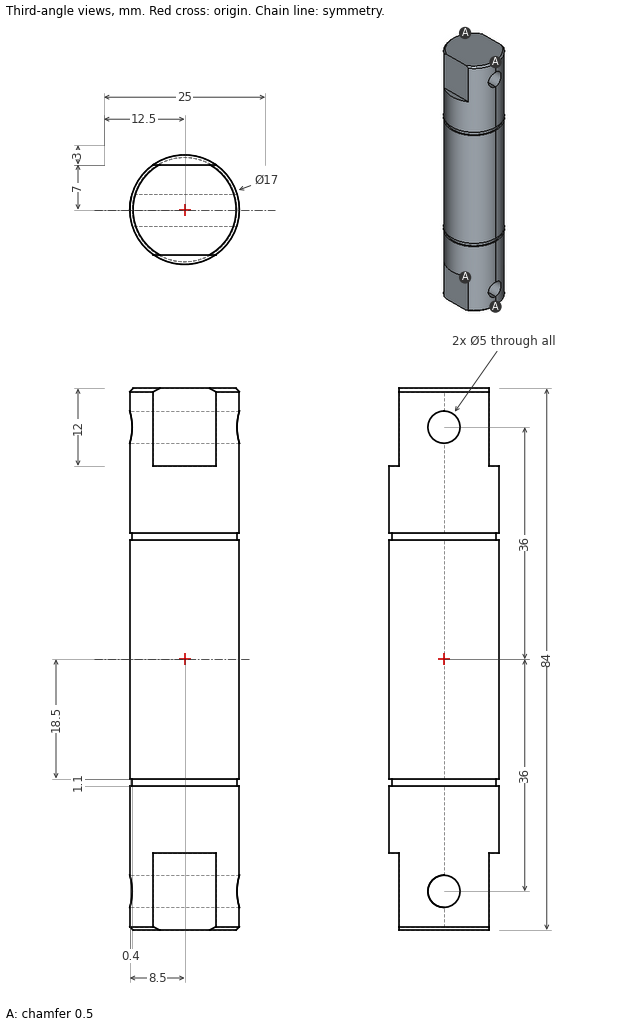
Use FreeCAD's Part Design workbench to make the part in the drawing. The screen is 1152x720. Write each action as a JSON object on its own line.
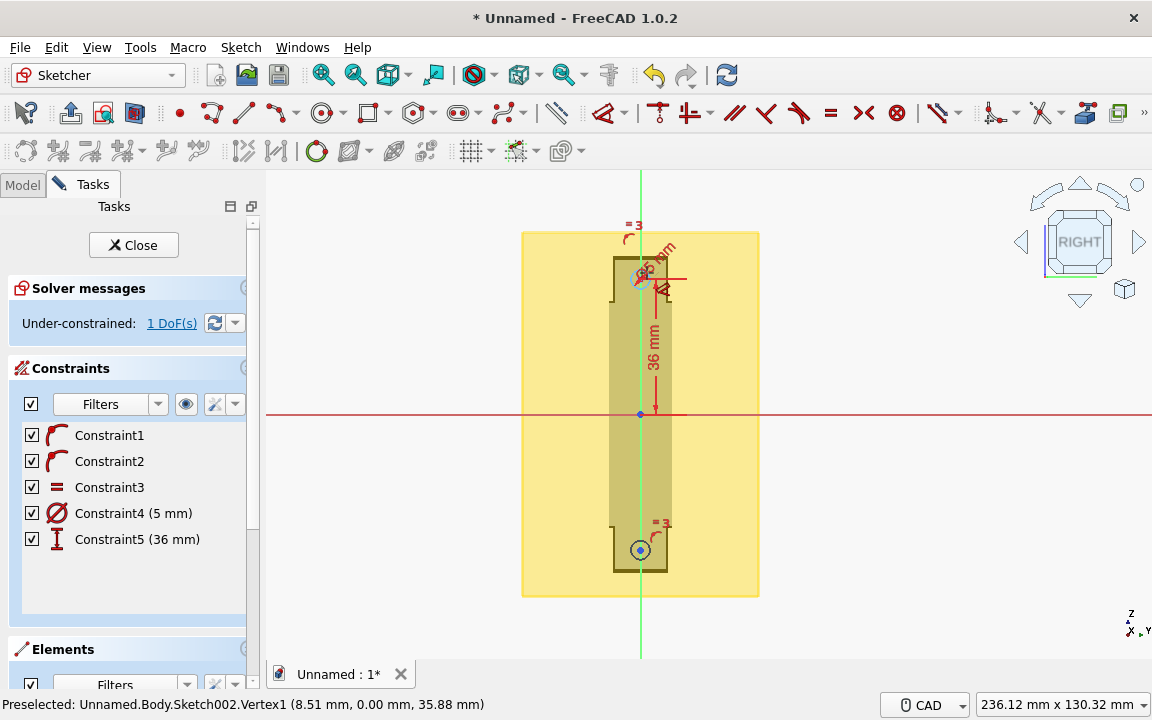
{"action": "left_click", "coordinate": [641, 550]}
{"action": "left_click", "coordinate": [675, 482]}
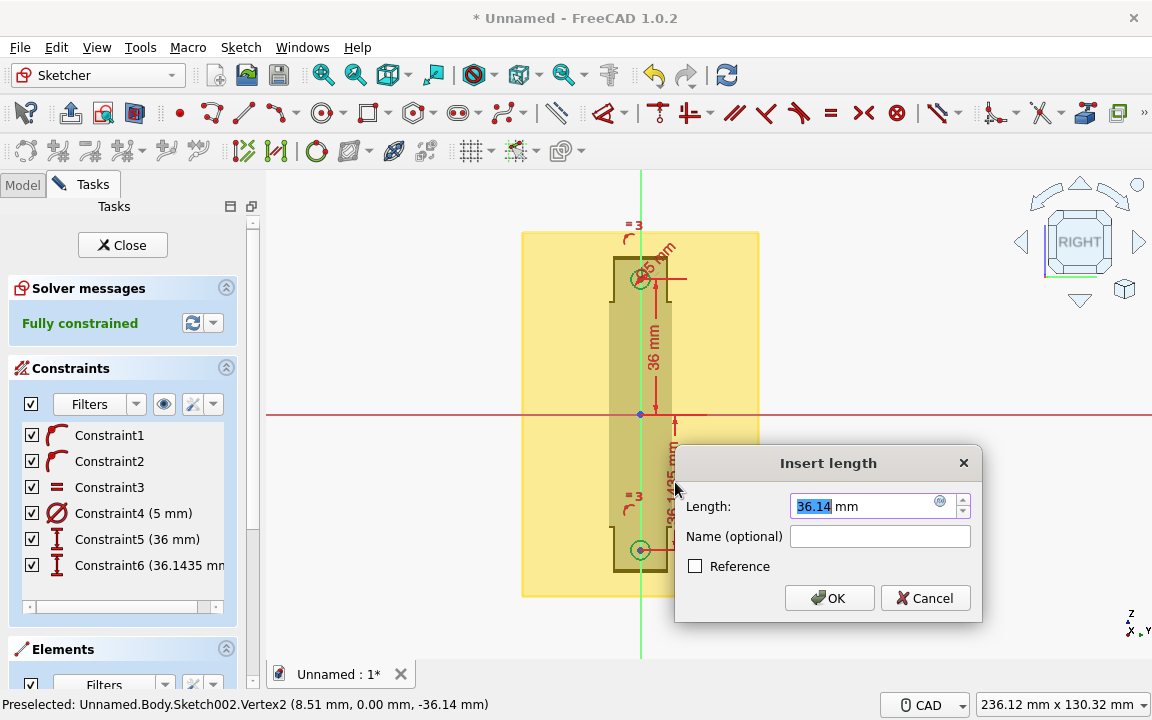
{"action": "type", "text": "36"}
{"action": "key", "text": "Return"}
{"action": "key", "text": "Escape"}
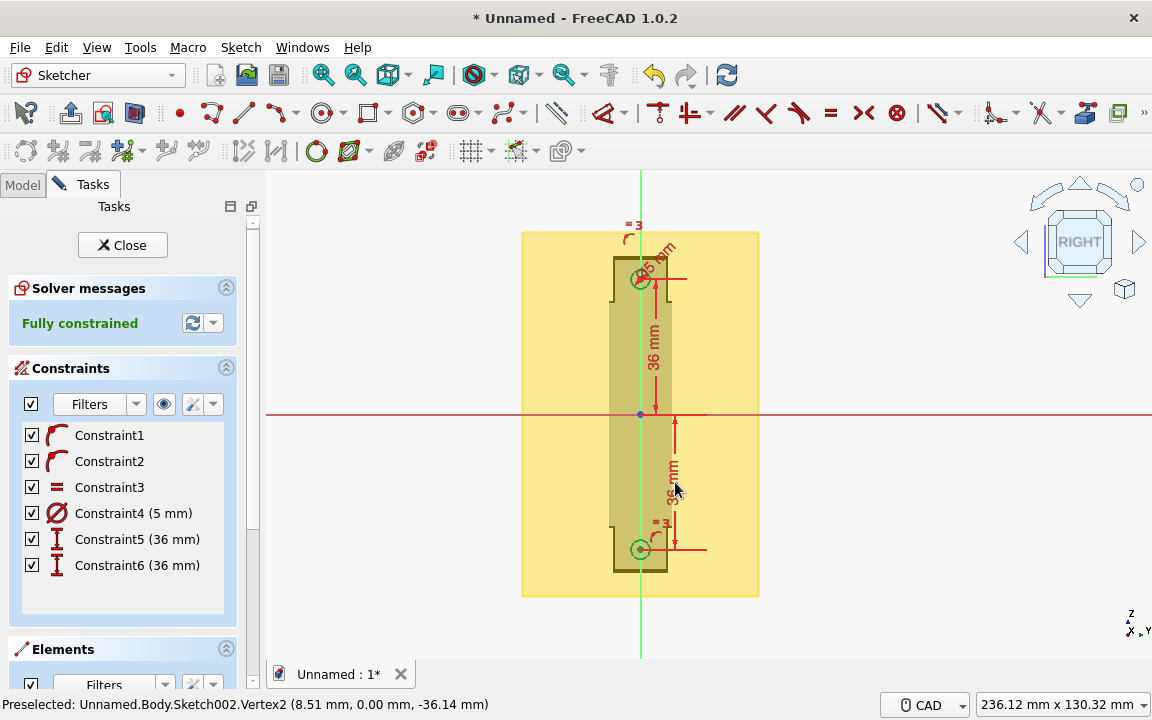
{"action": "left_click", "coordinate": [123, 245]}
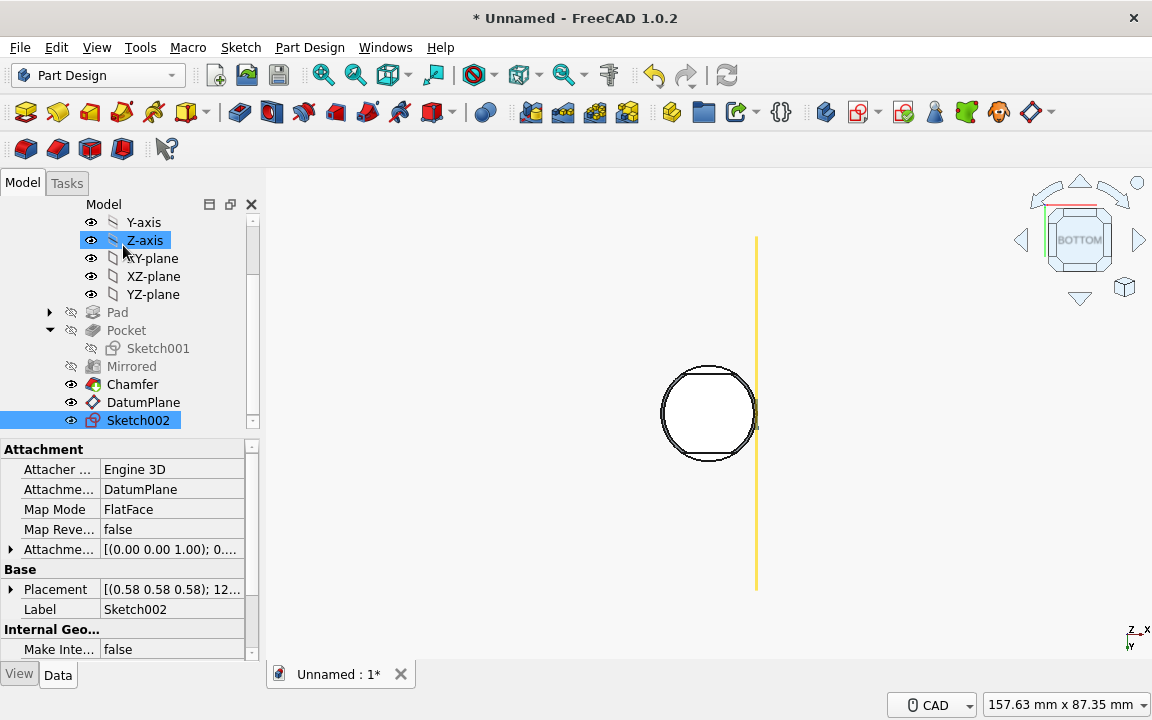
{"action": "left_click", "coordinate": [272, 112]}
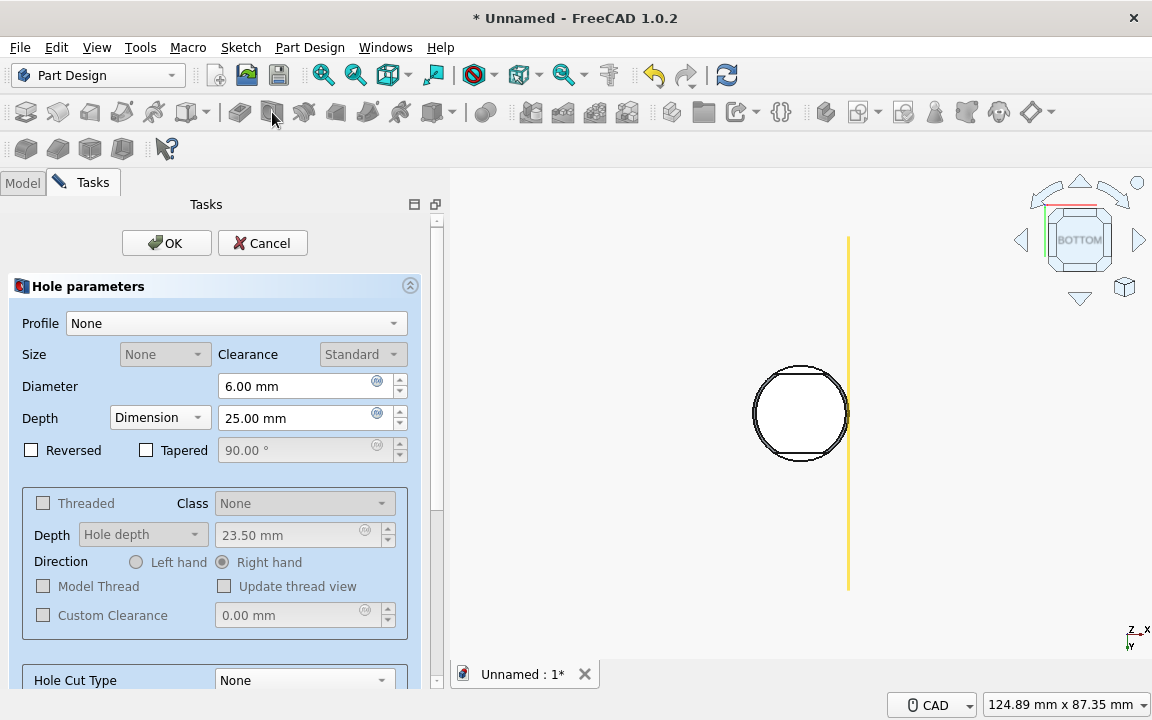
{"action": "triple_click", "coordinate": [305, 386]}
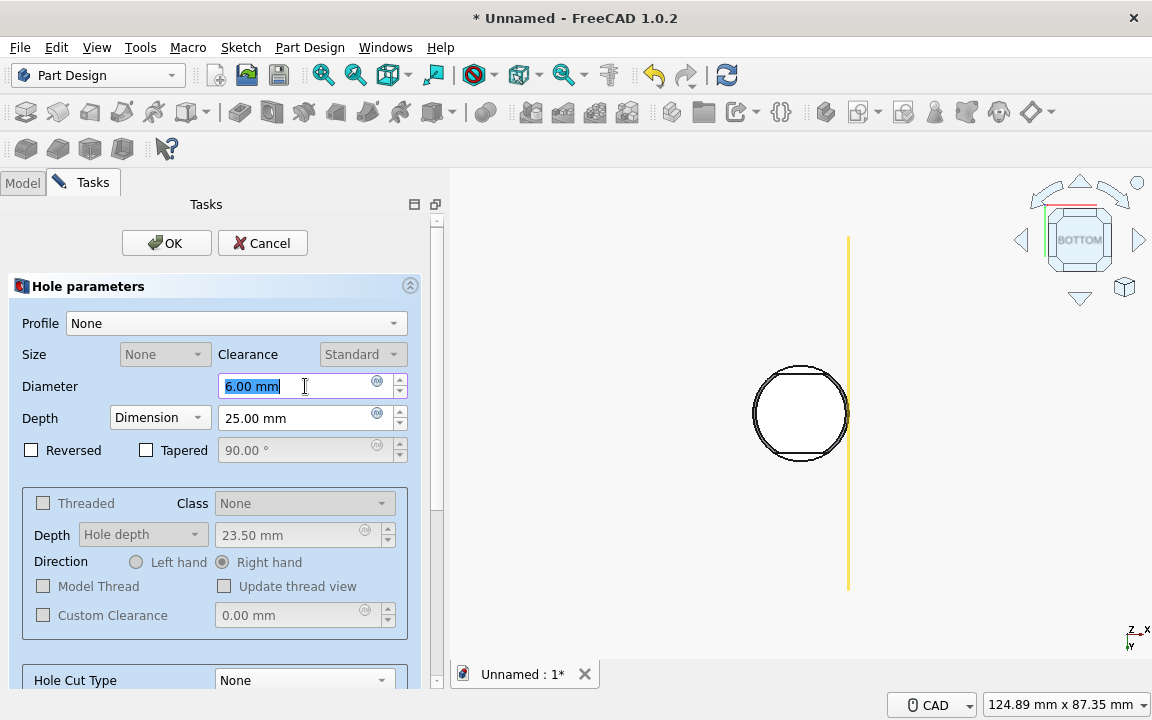
{"action": "type", "text": "5"}
{"action": "key", "text": "Tab"}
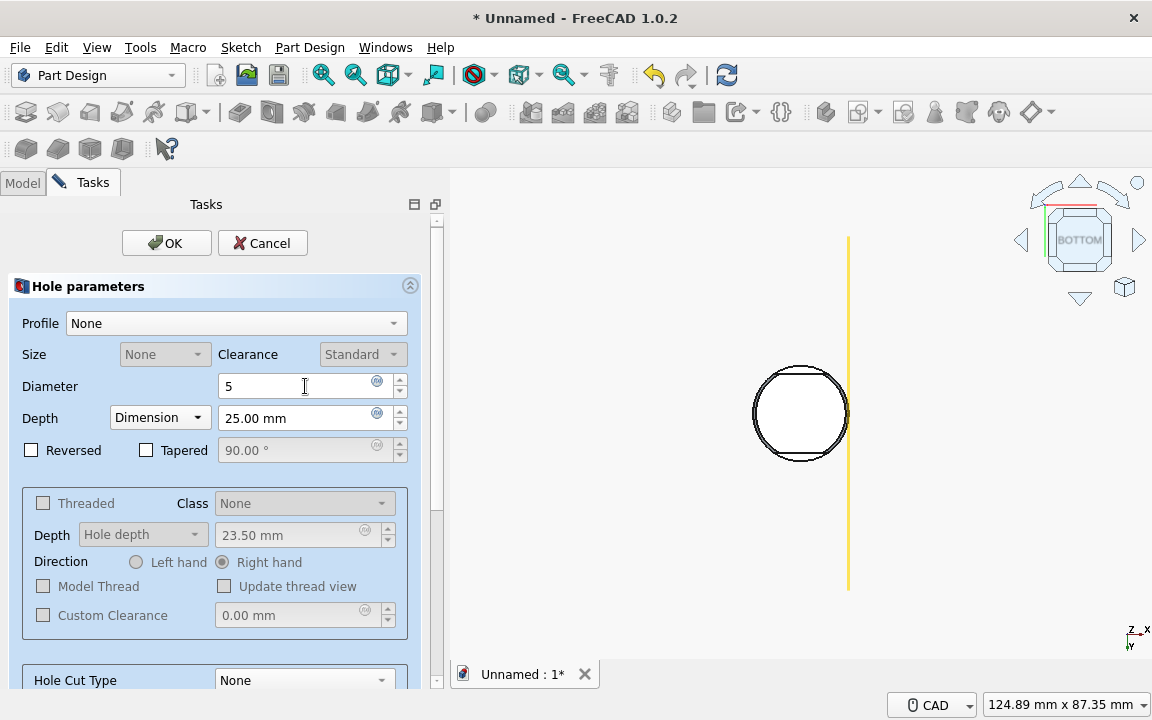
{"action": "left_click", "coordinate": [161, 418]}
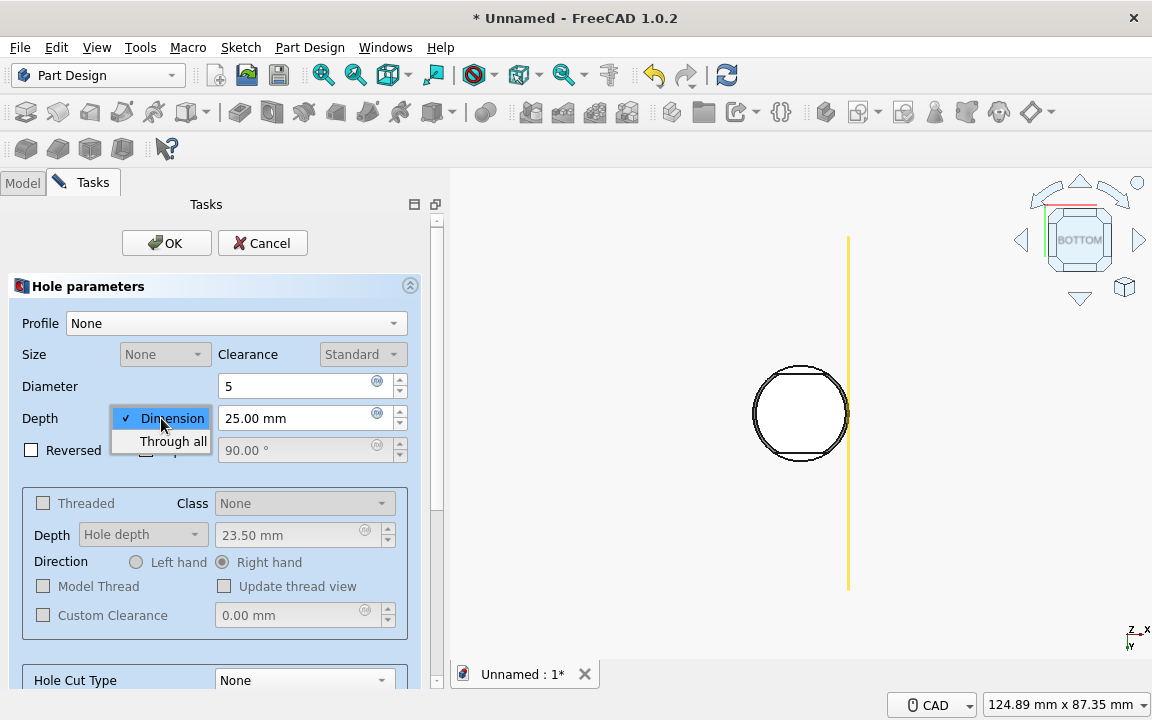
{"action": "left_click", "coordinate": [160, 442]}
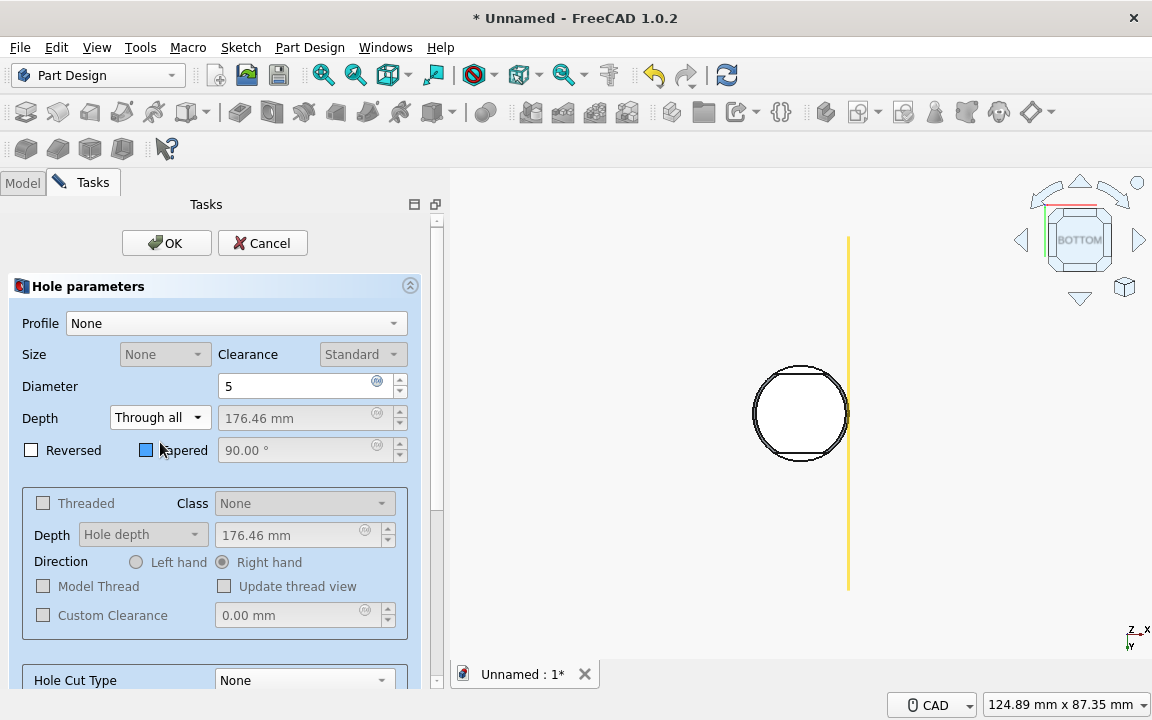
{"action": "left_click", "coordinate": [167, 243]}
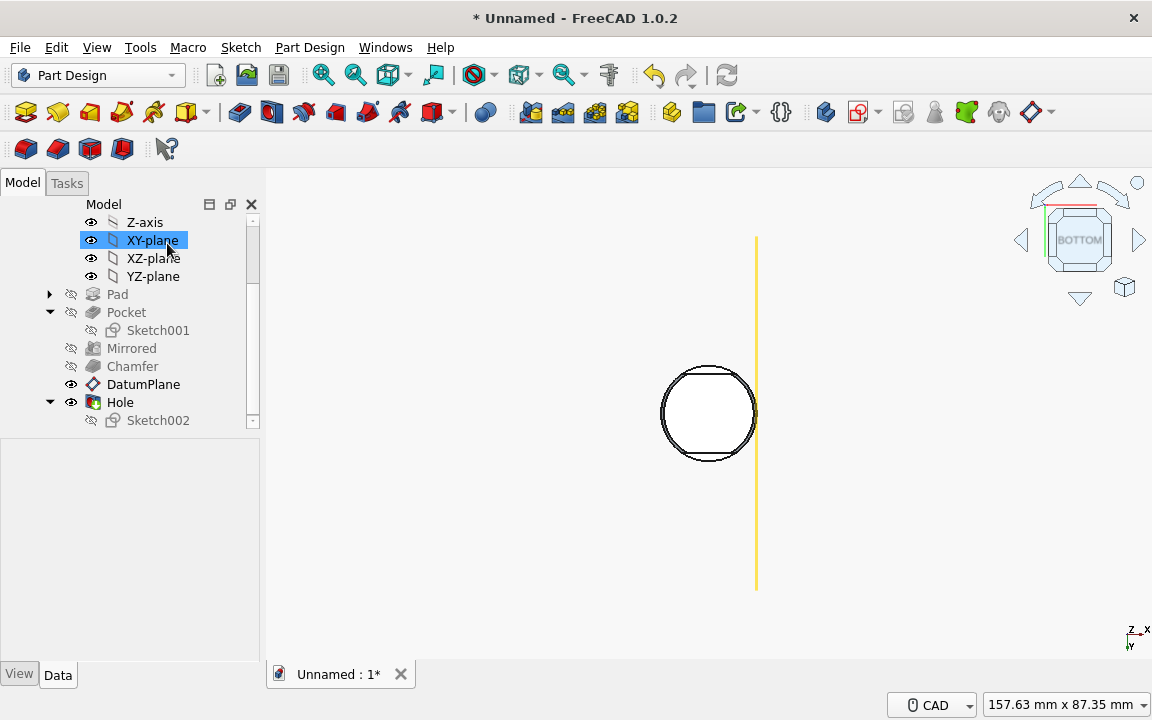
{"action": "left_click", "coordinate": [116, 384]}
{"action": "key", "text": "space"}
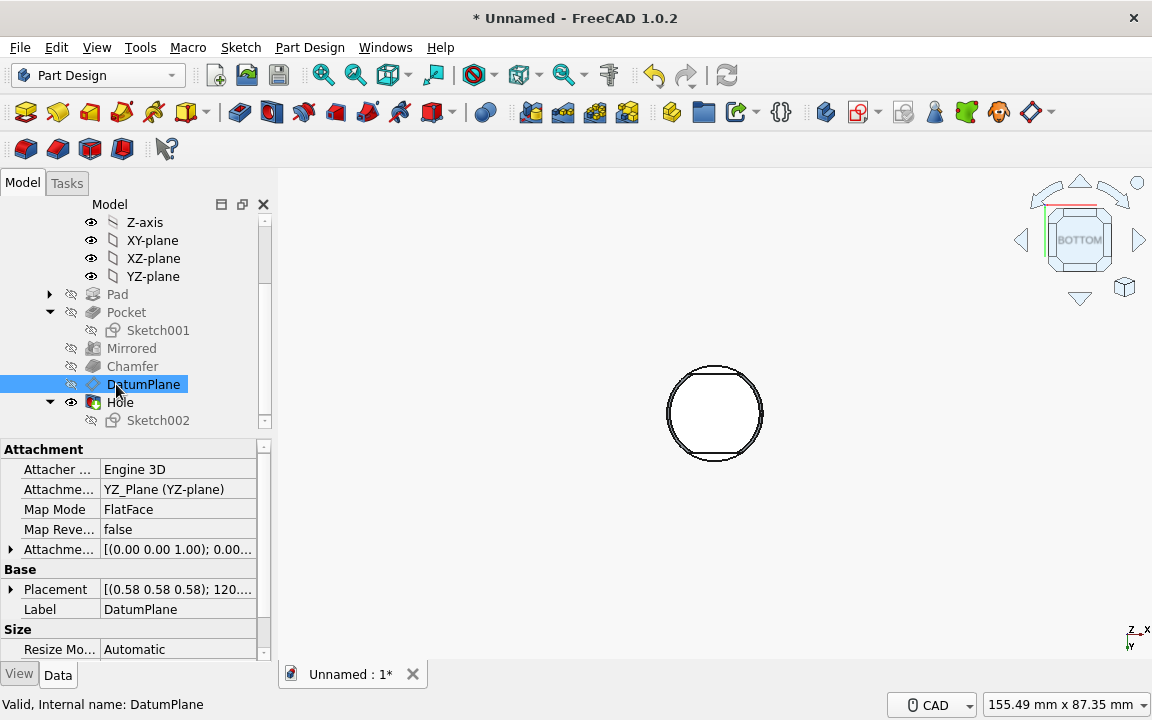
{"action": "left_click", "coordinate": [324, 76]}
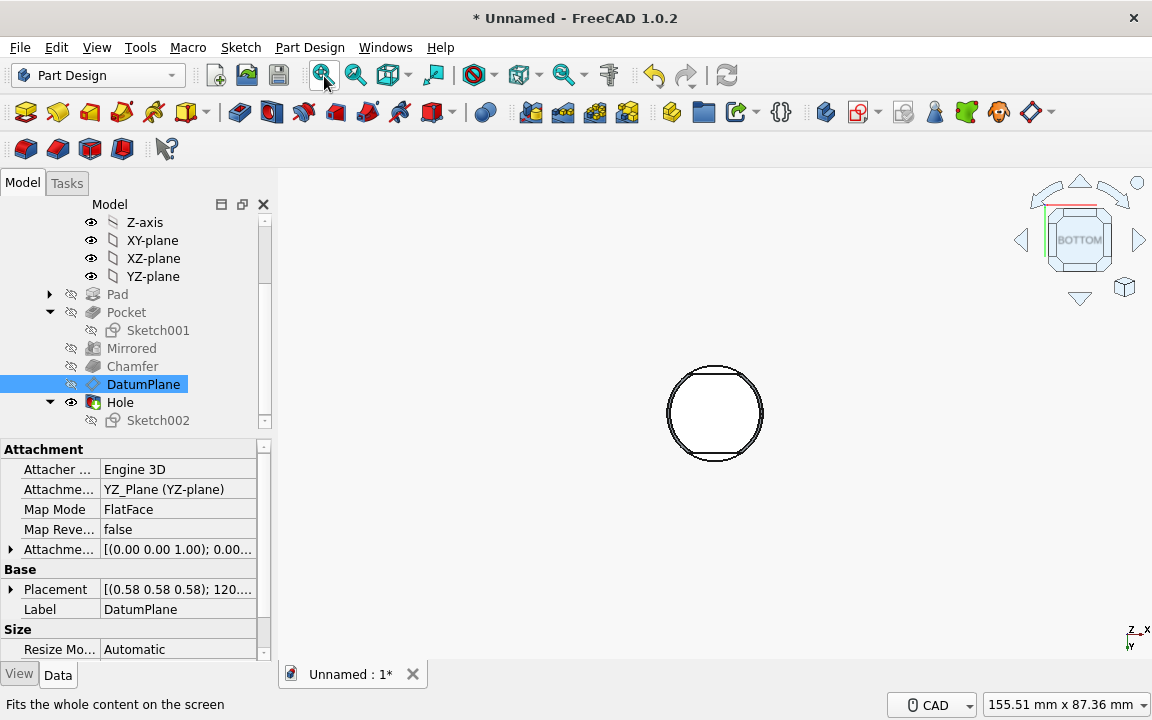
{"action": "left_click", "coordinate": [318, 619]}